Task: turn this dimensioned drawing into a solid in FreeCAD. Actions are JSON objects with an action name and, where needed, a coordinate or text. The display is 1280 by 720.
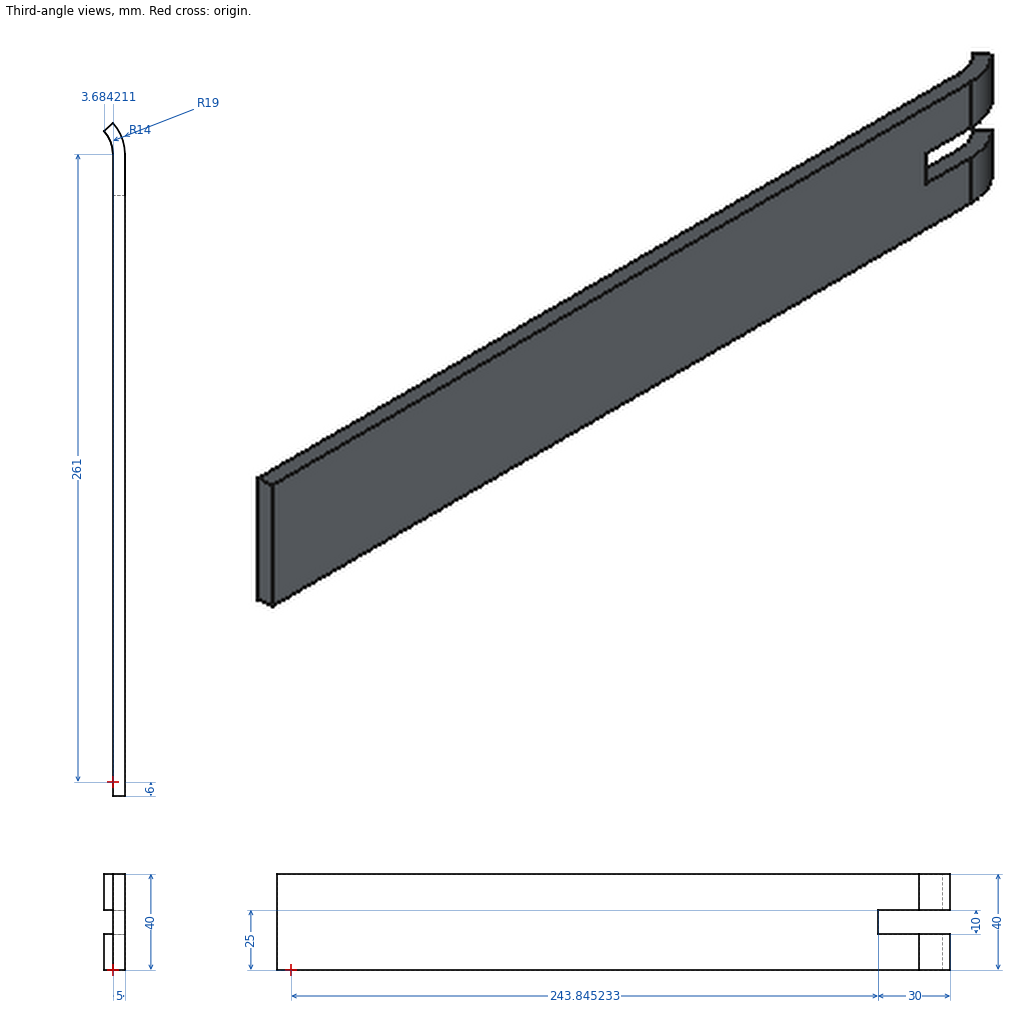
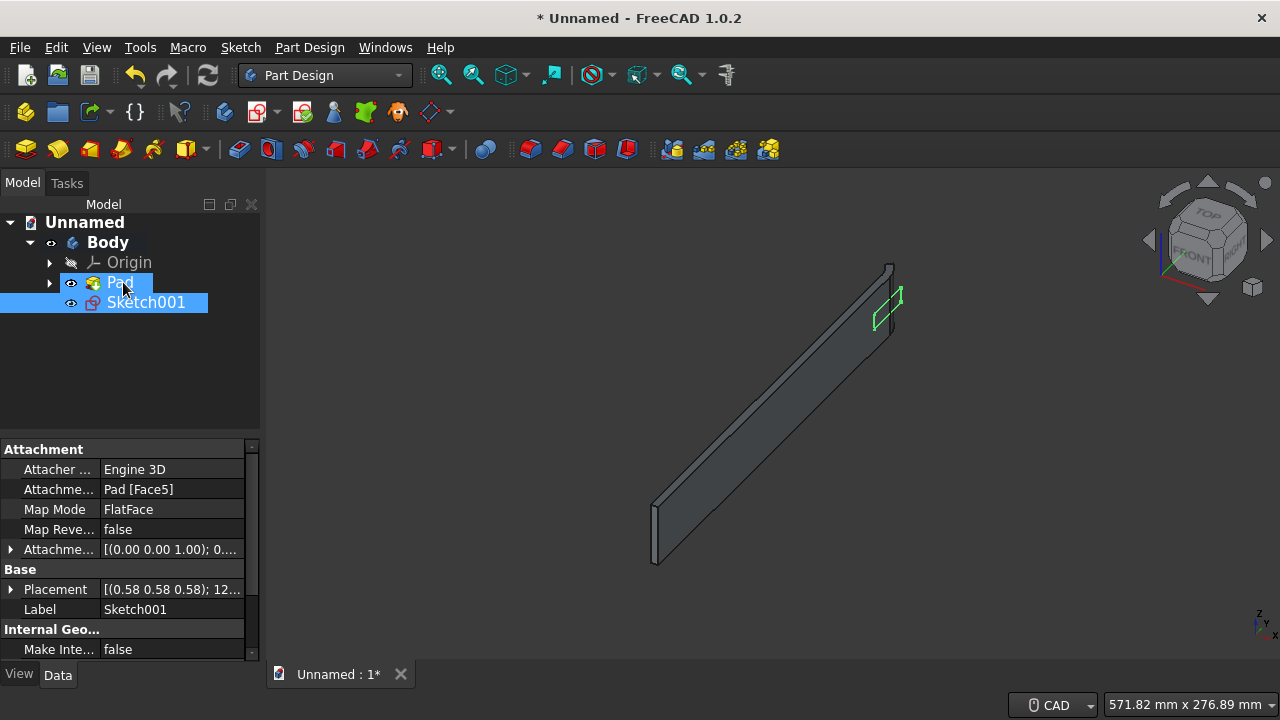
{"action": "left_click", "coordinate": [240, 150]}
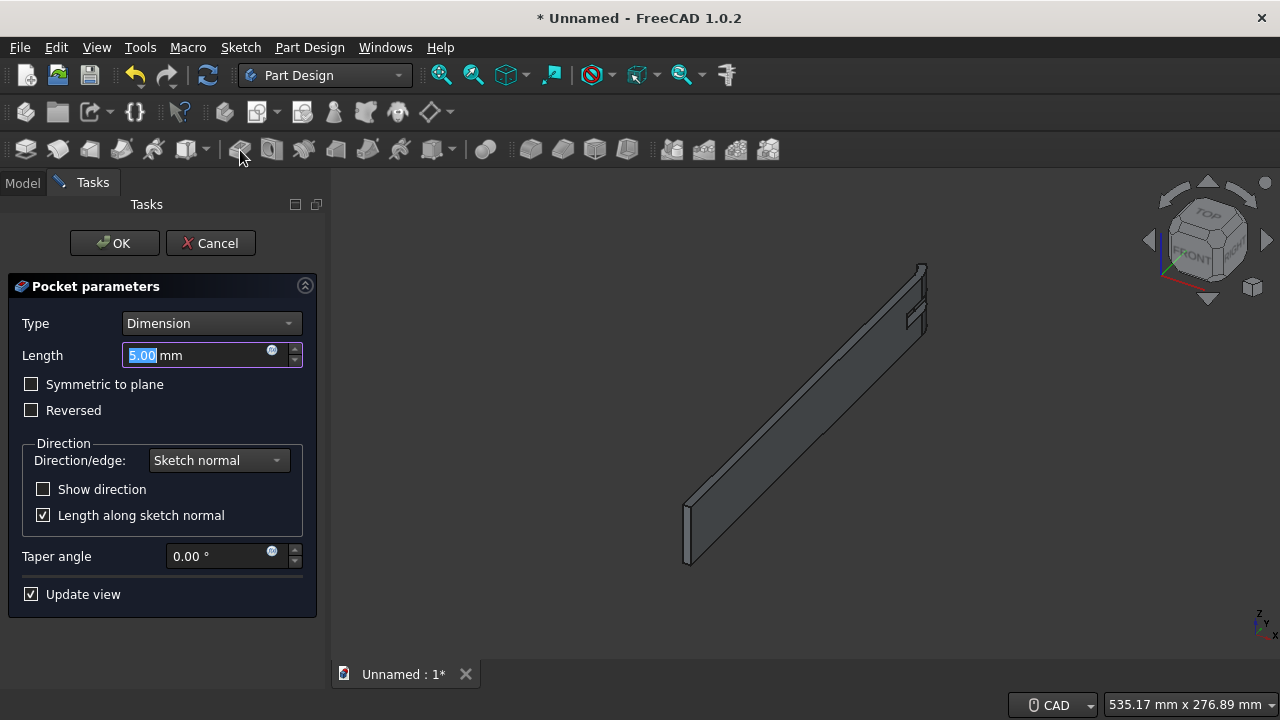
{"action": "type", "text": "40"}
{"action": "key", "text": "Tab"}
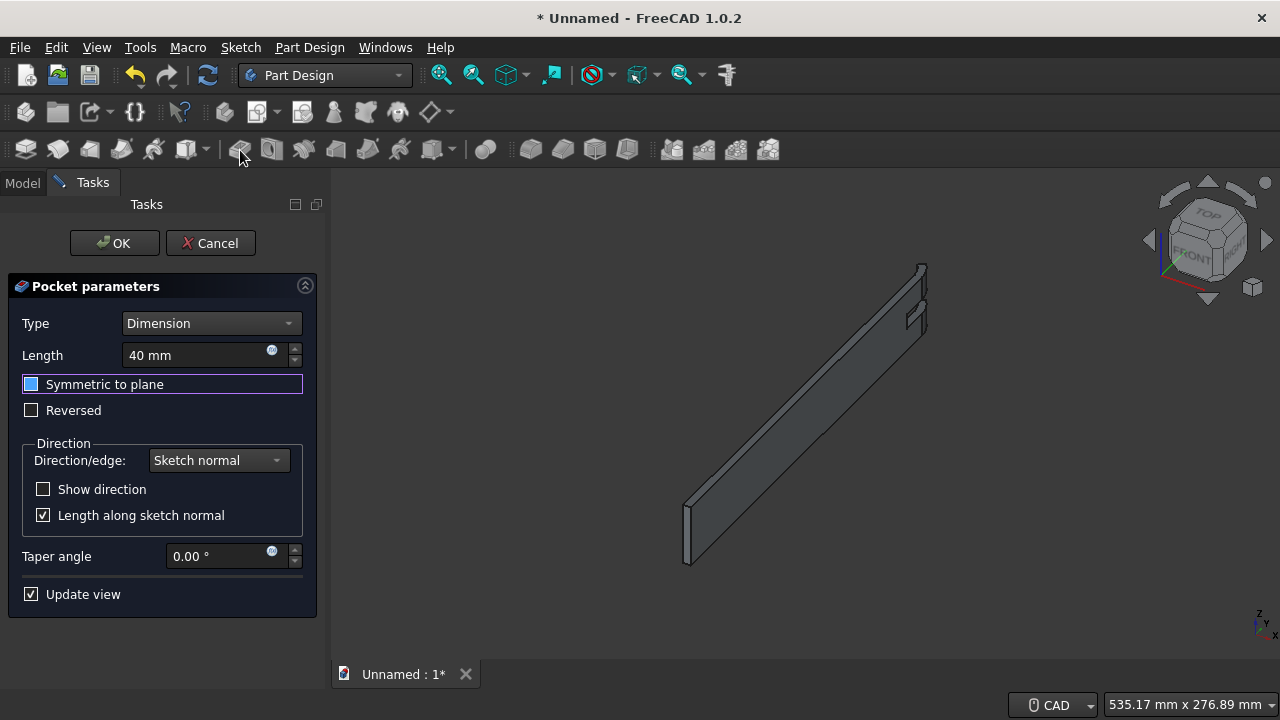
{"action": "left_click", "coordinate": [115, 243]}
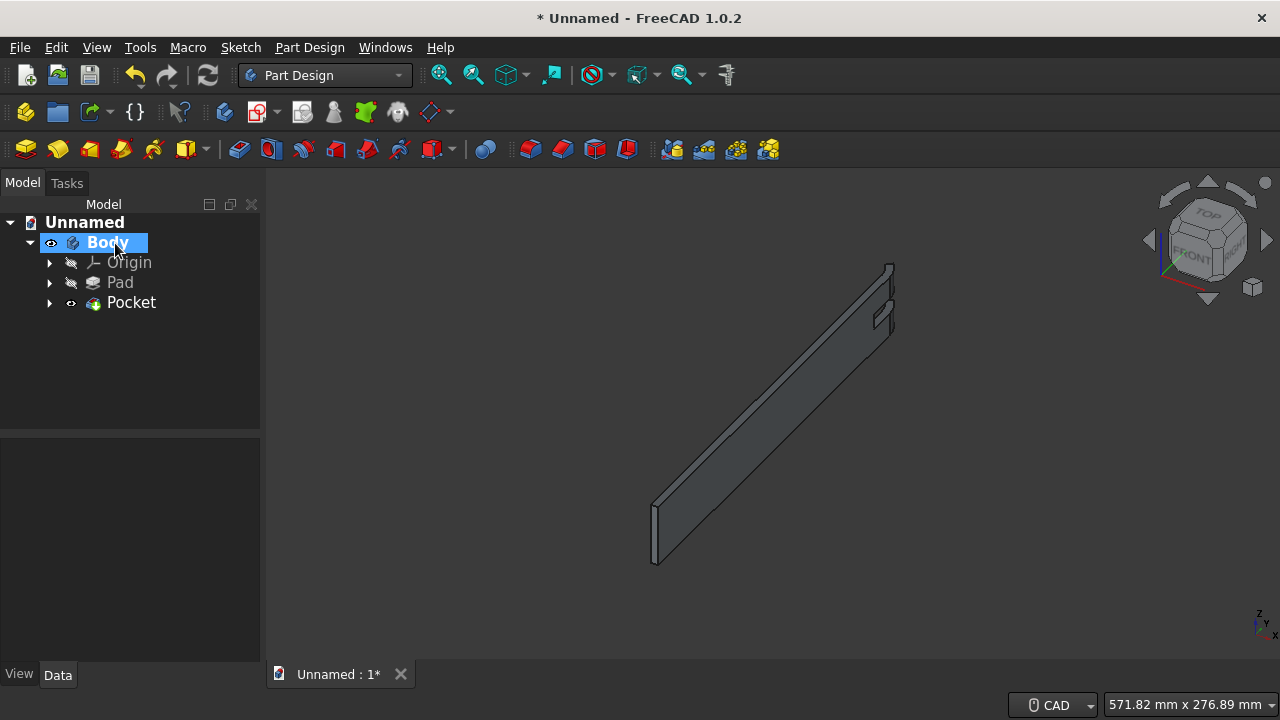
{"action": "scroll", "coordinate": [654, 509], "scroll_direction": "up", "scroll_amount": 5}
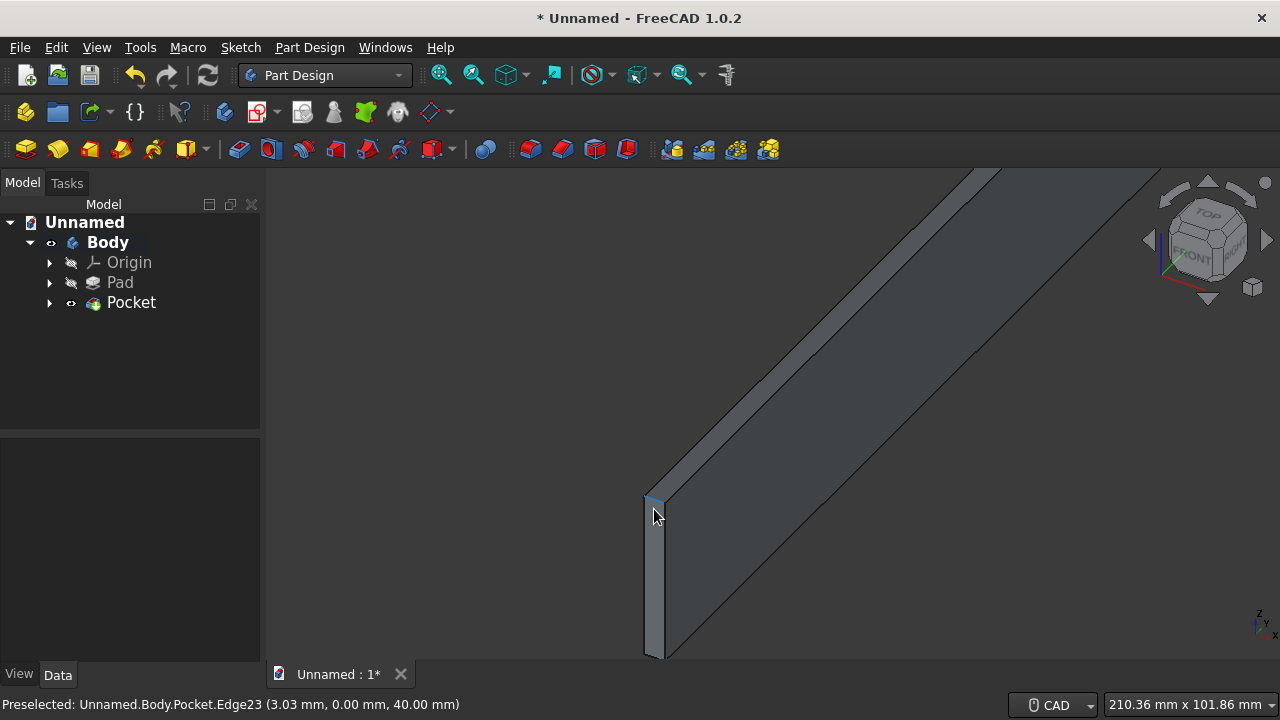
{"action": "left_click", "coordinate": [655, 510]}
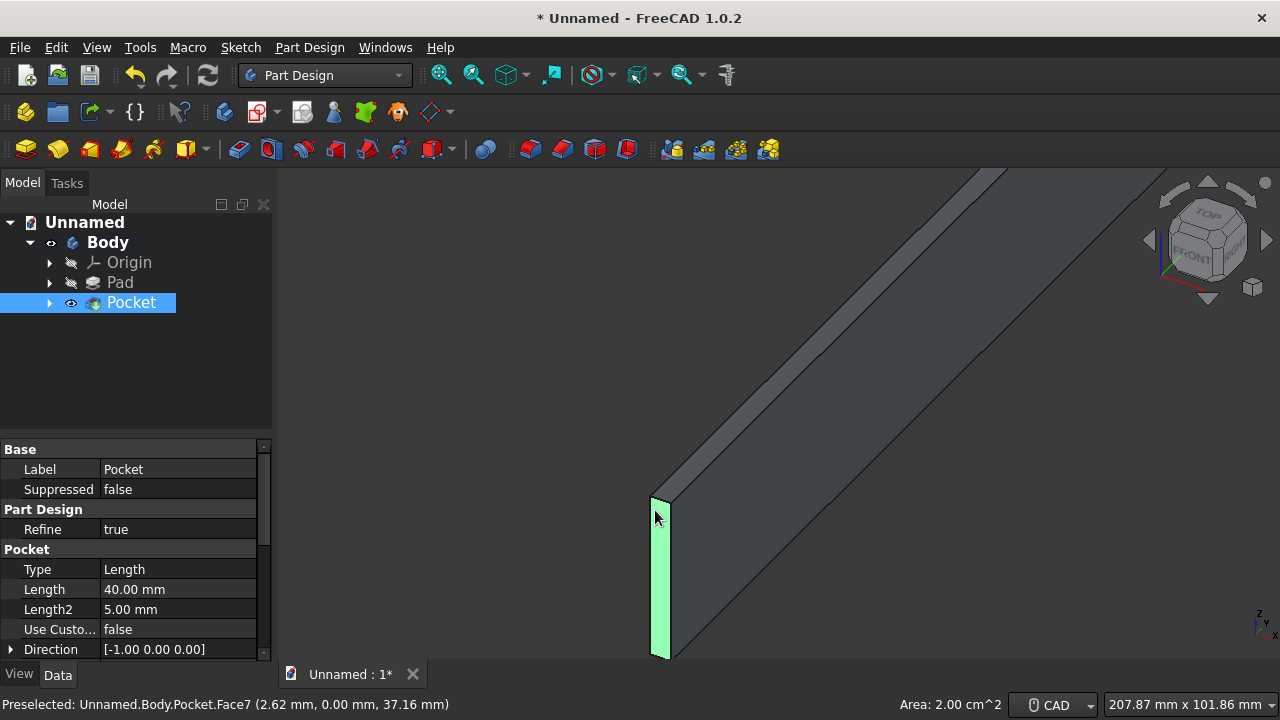
{"action": "left_click", "coordinate": [258, 112]}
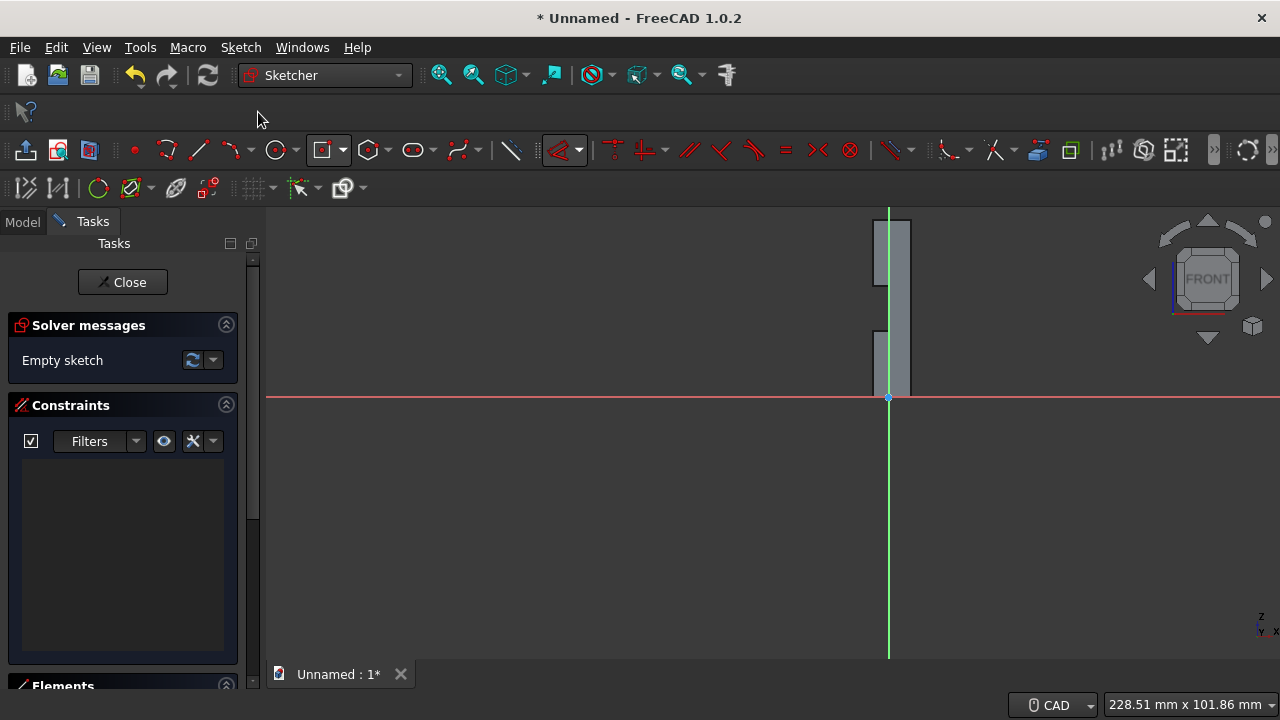
{"action": "scroll", "coordinate": [294, 631], "scroll_direction": "down", "scroll_amount": 1}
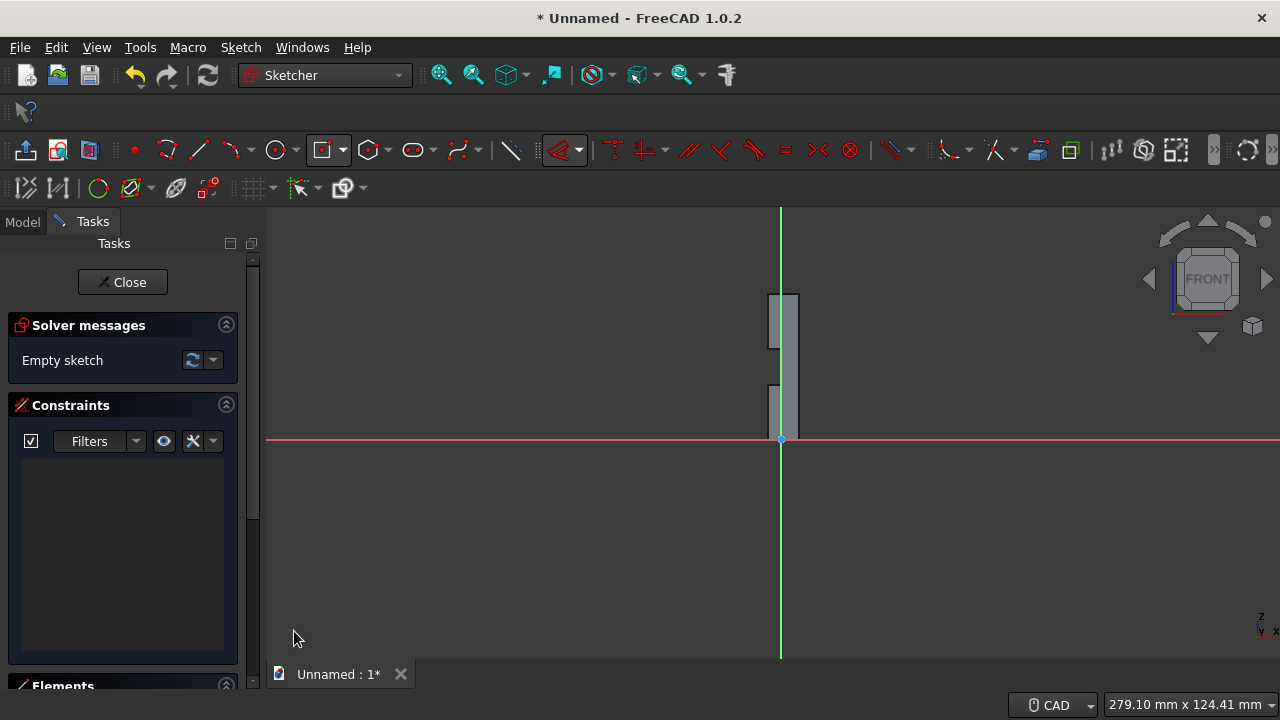
{"action": "scroll", "coordinate": [894, 287], "scroll_direction": "up", "scroll_amount": 3}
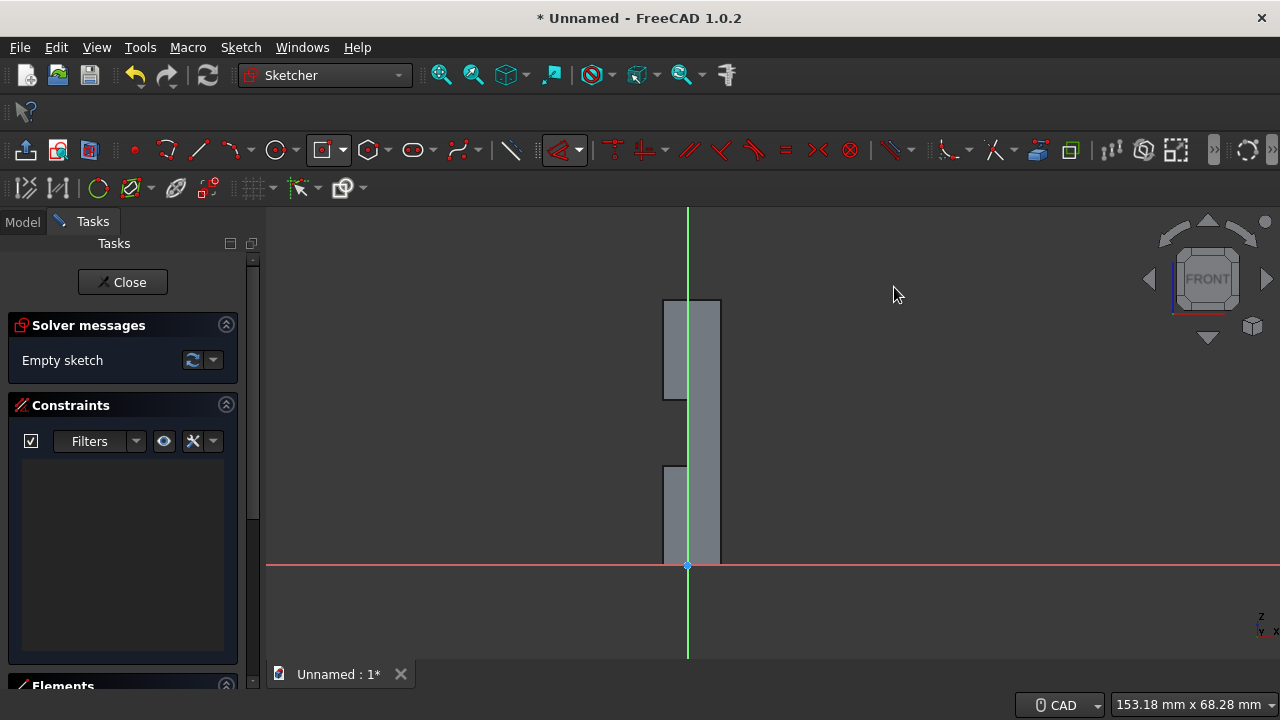
{"action": "left_click", "coordinate": [346, 150]}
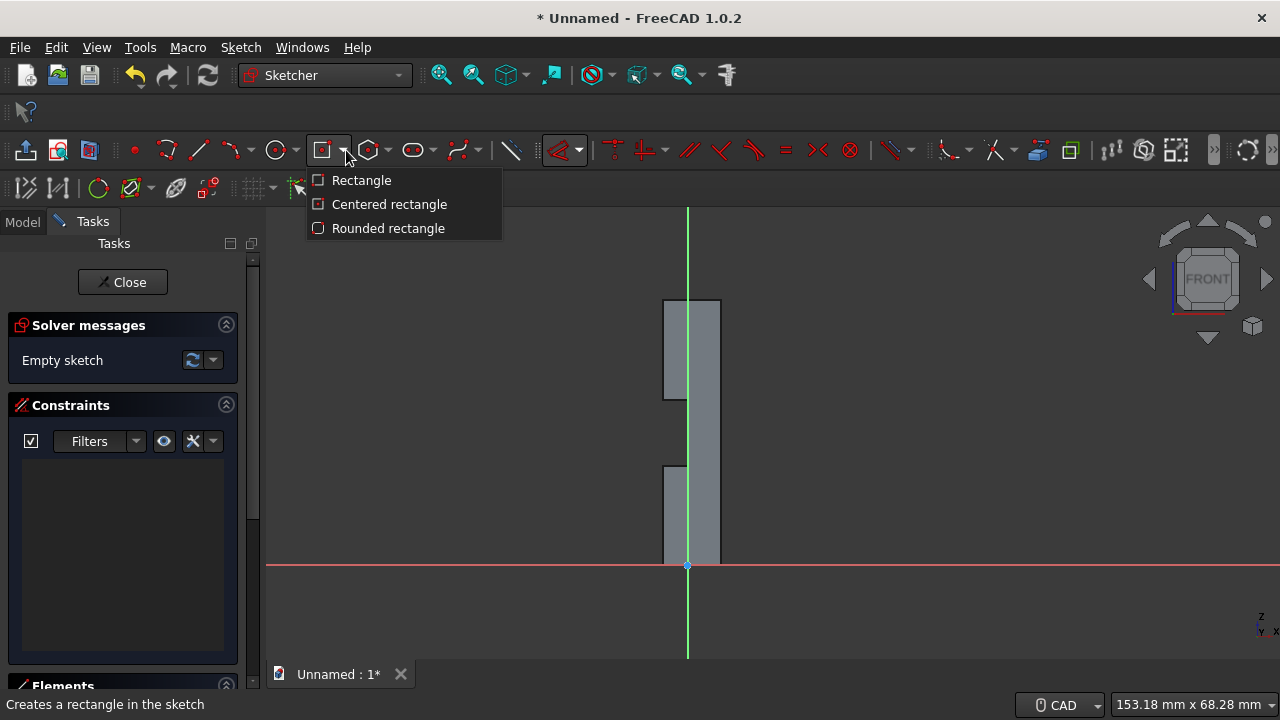
{"action": "left_click", "coordinate": [404, 180]}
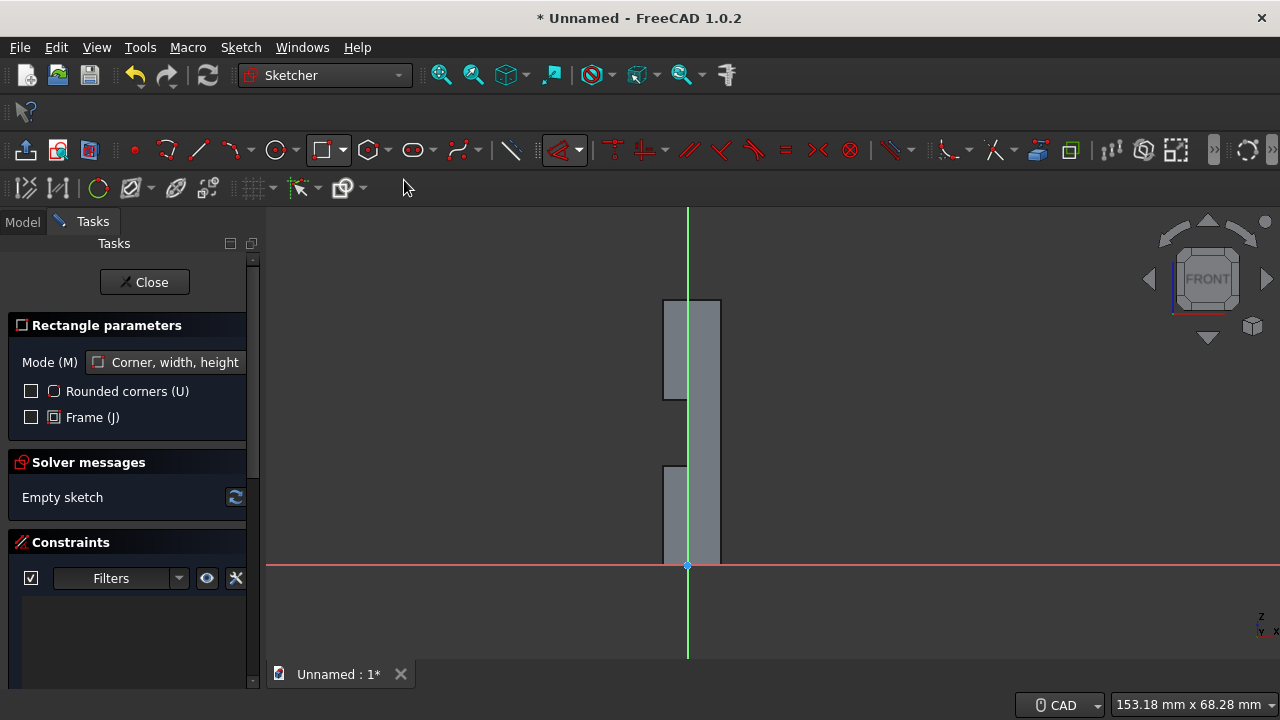
{"action": "left_click", "coordinate": [688, 565]}
{"action": "mouse_move", "coordinate": [721, 300]}